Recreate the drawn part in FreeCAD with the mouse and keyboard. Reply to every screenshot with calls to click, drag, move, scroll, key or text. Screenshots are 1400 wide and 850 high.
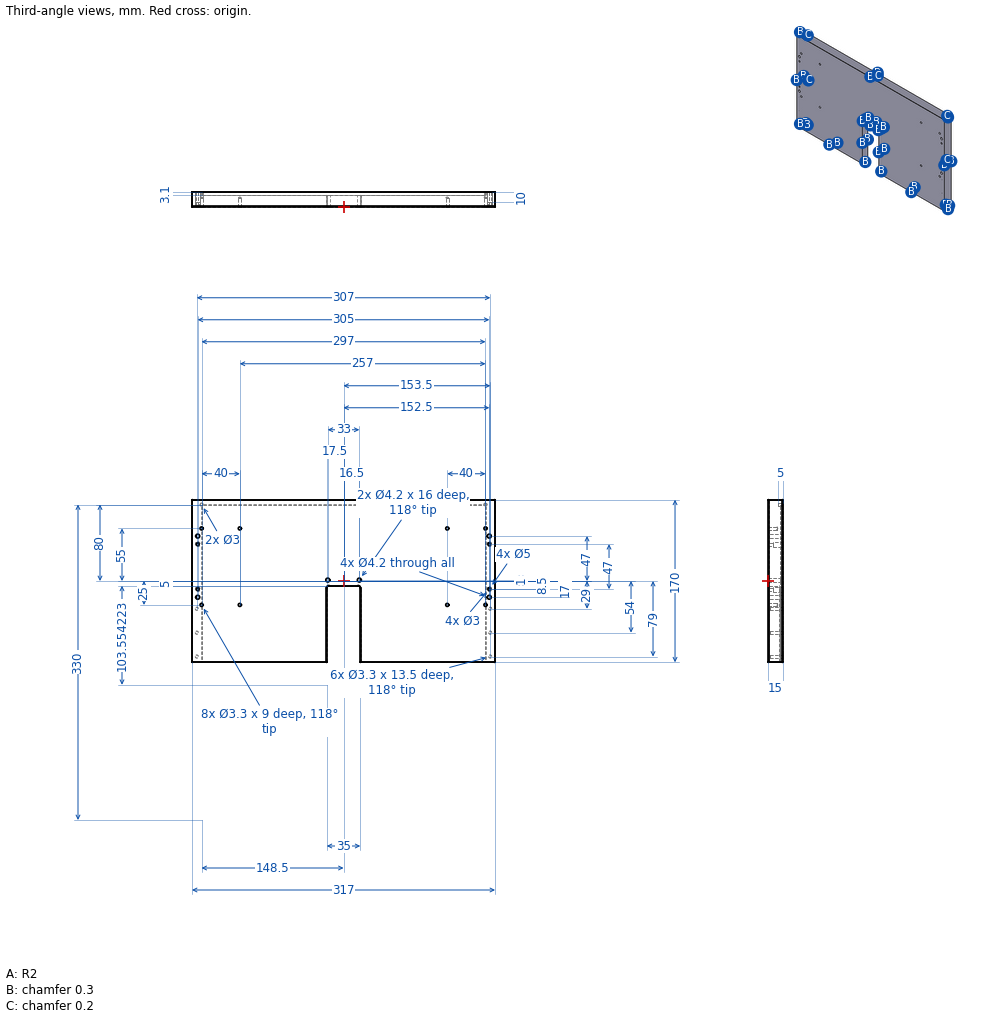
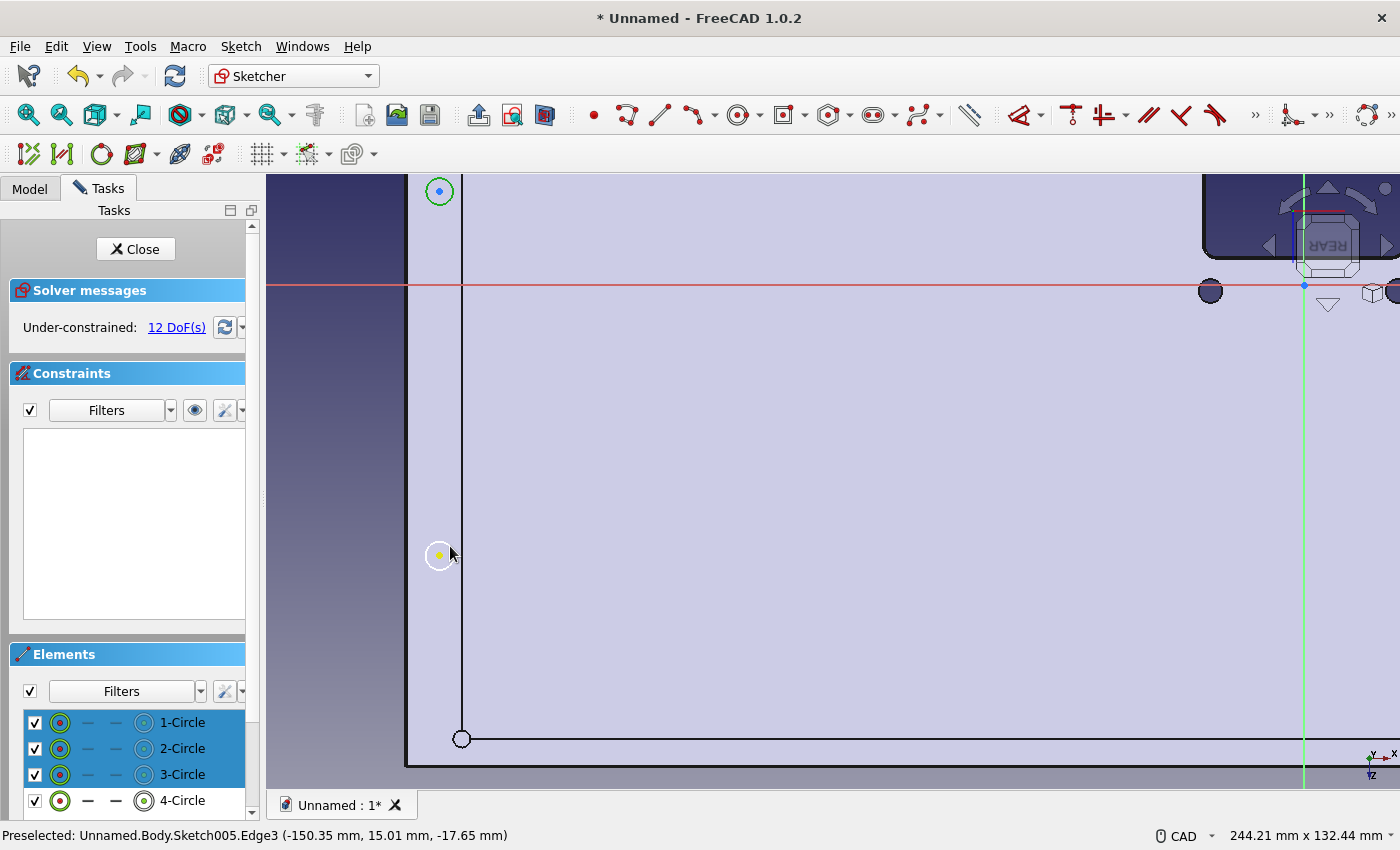
click(450, 546)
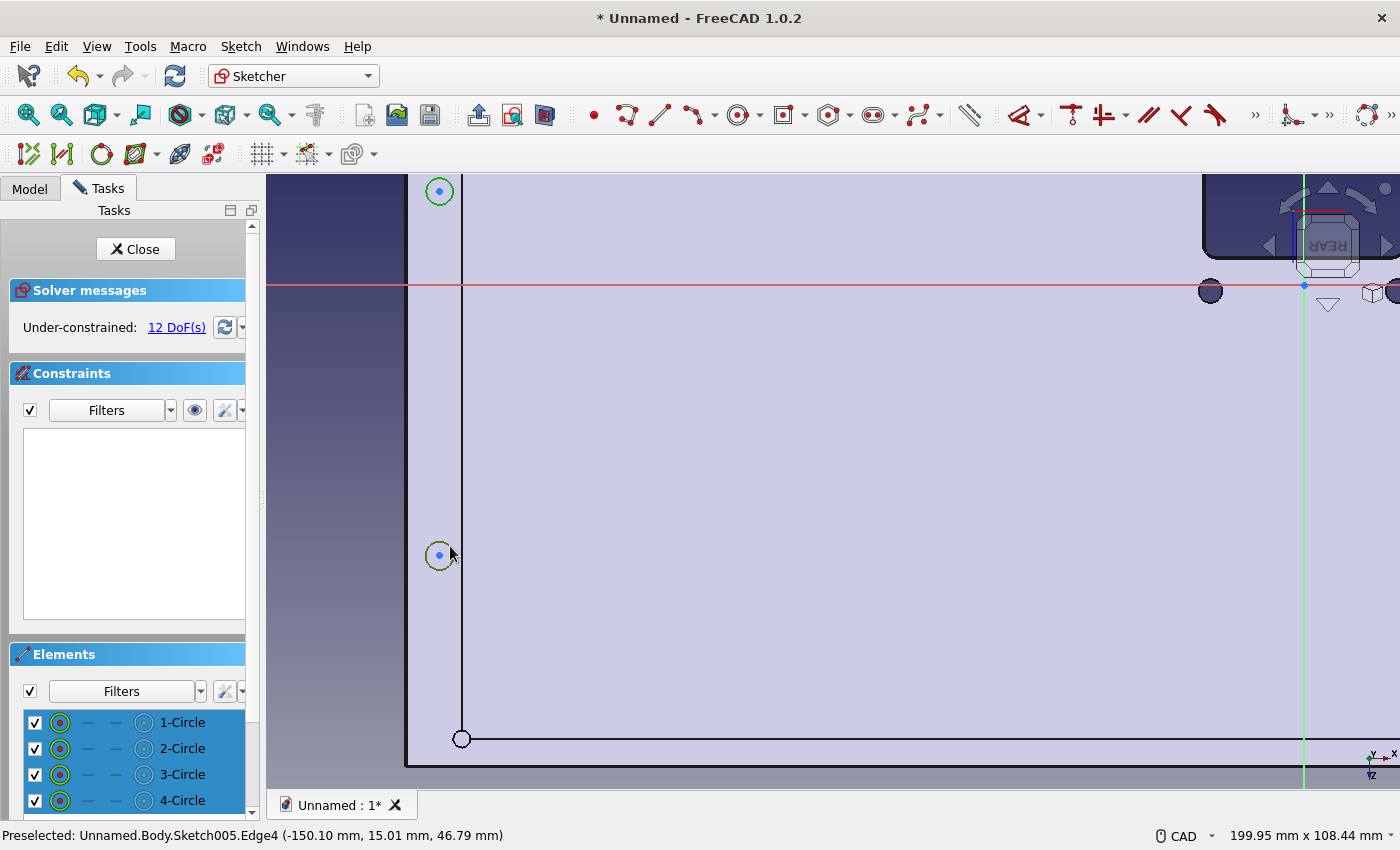
key(e)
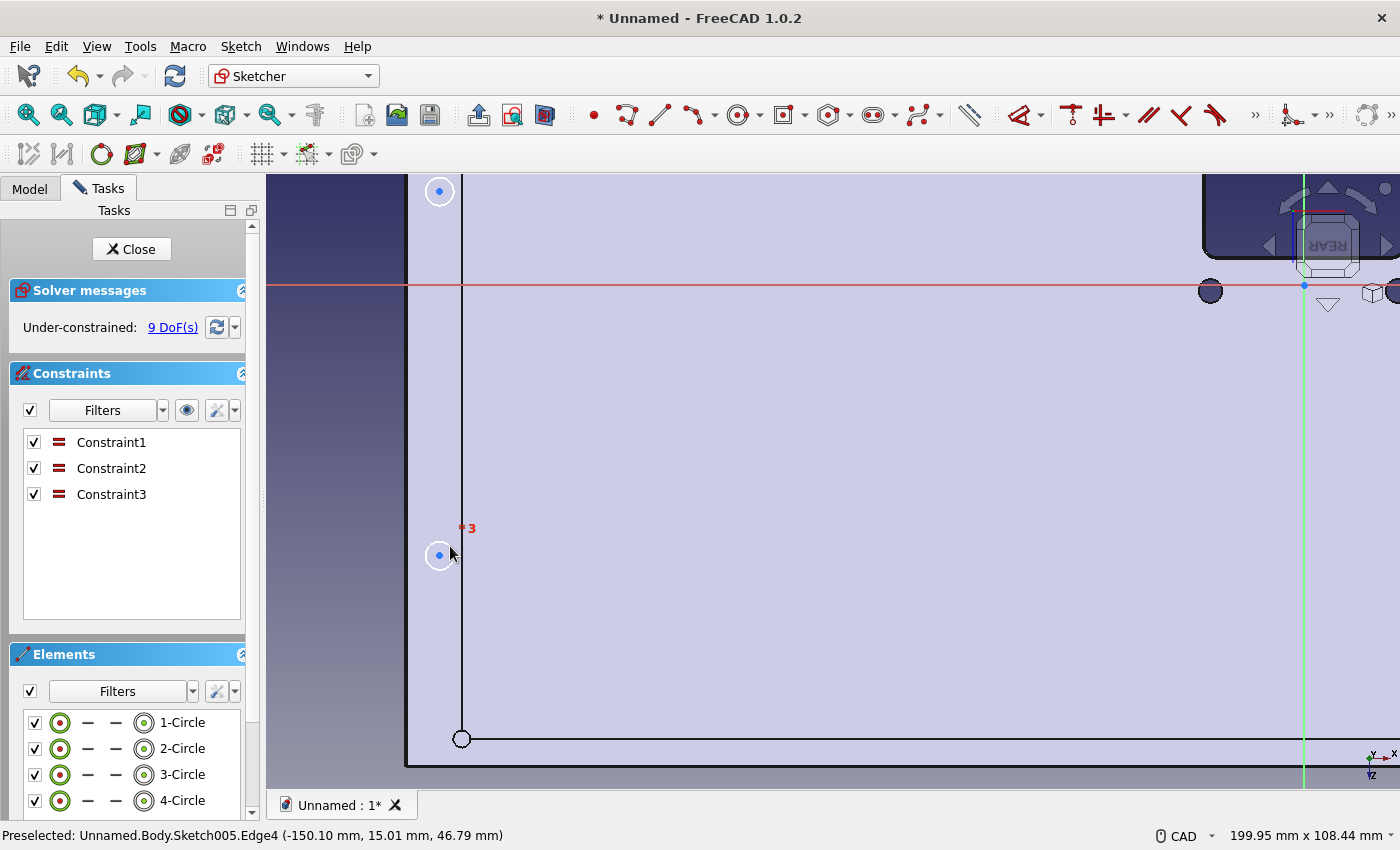
scroll(450, 546, down, 5)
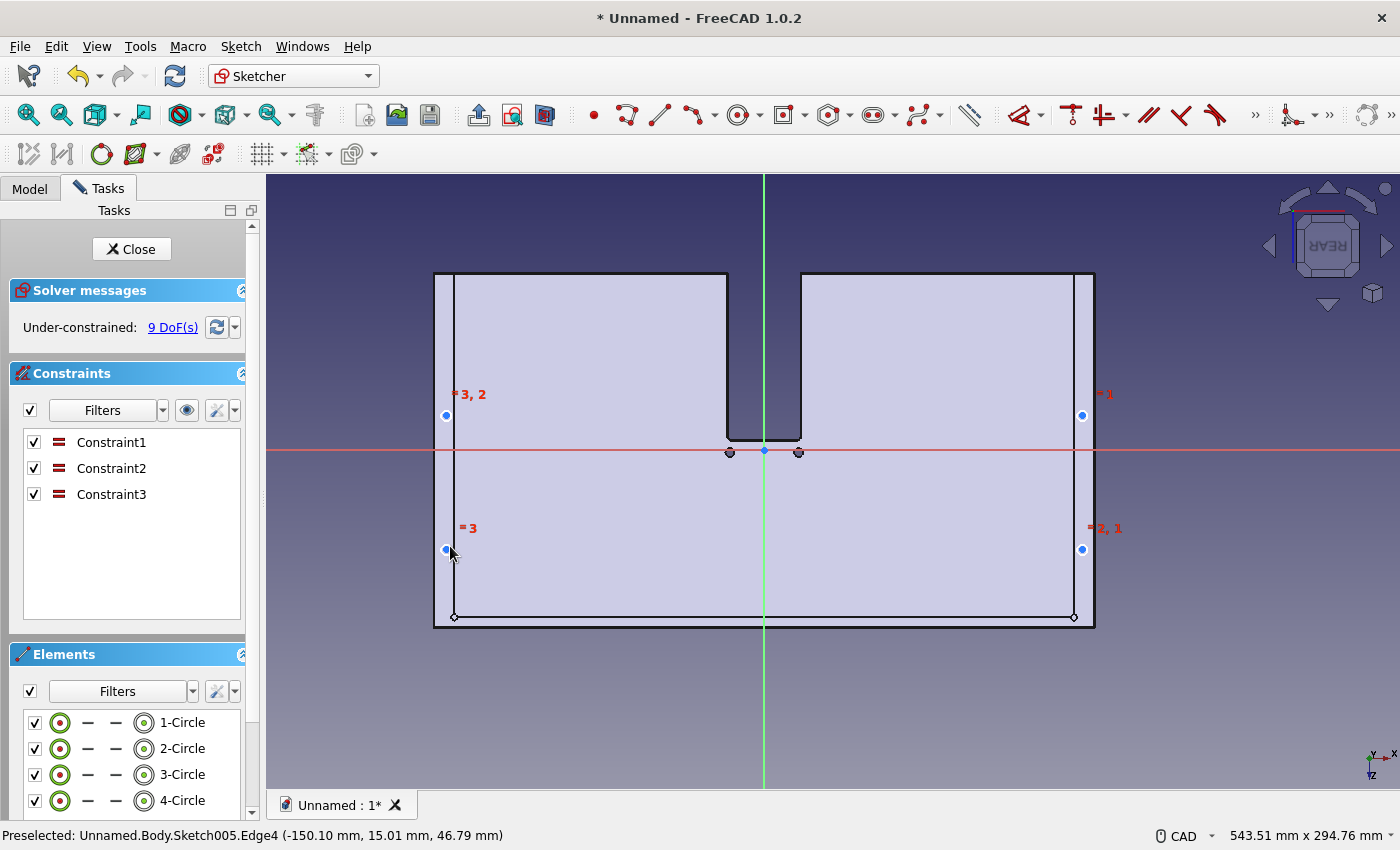
click(1082, 416)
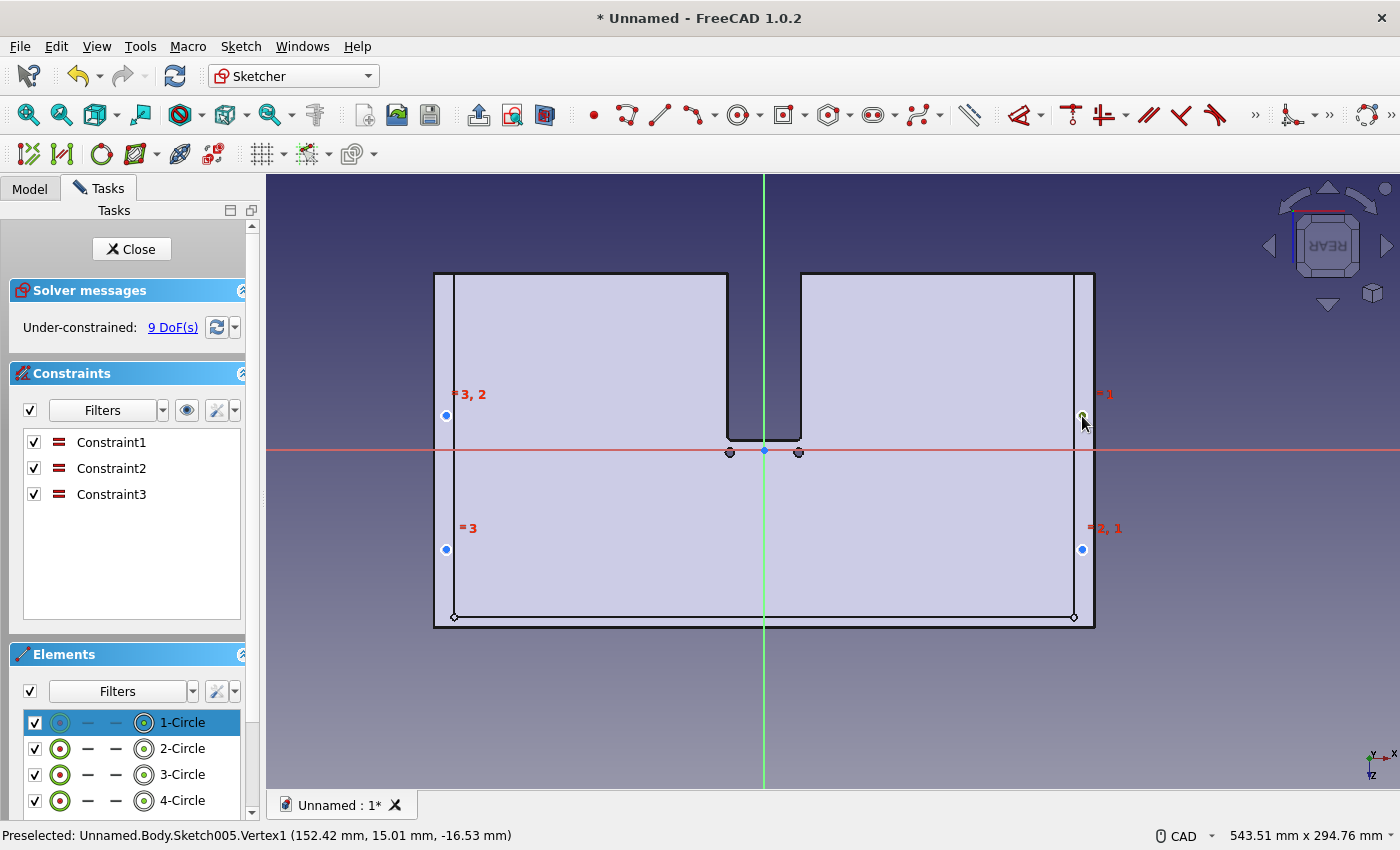
click(1082, 550)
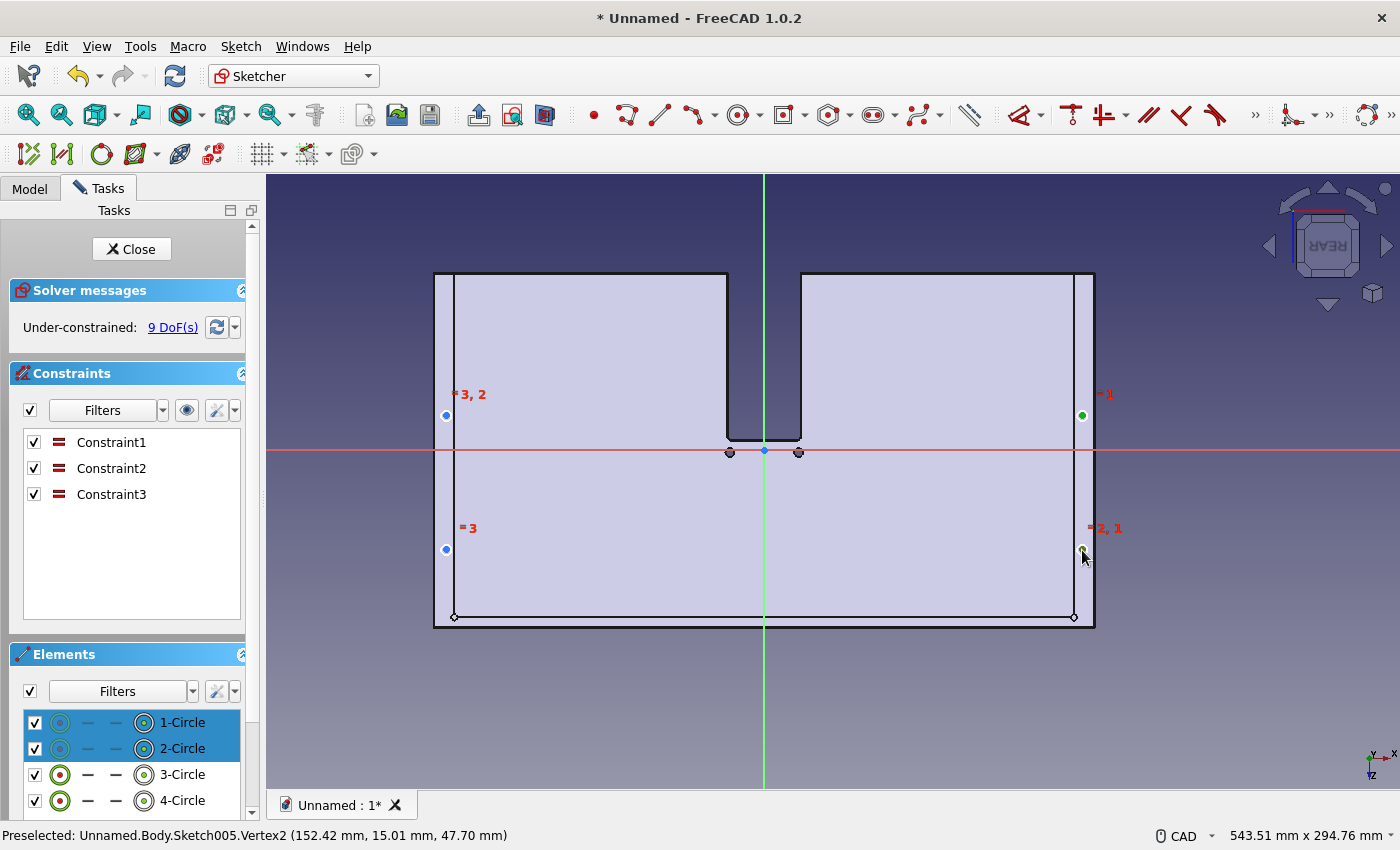
key(v)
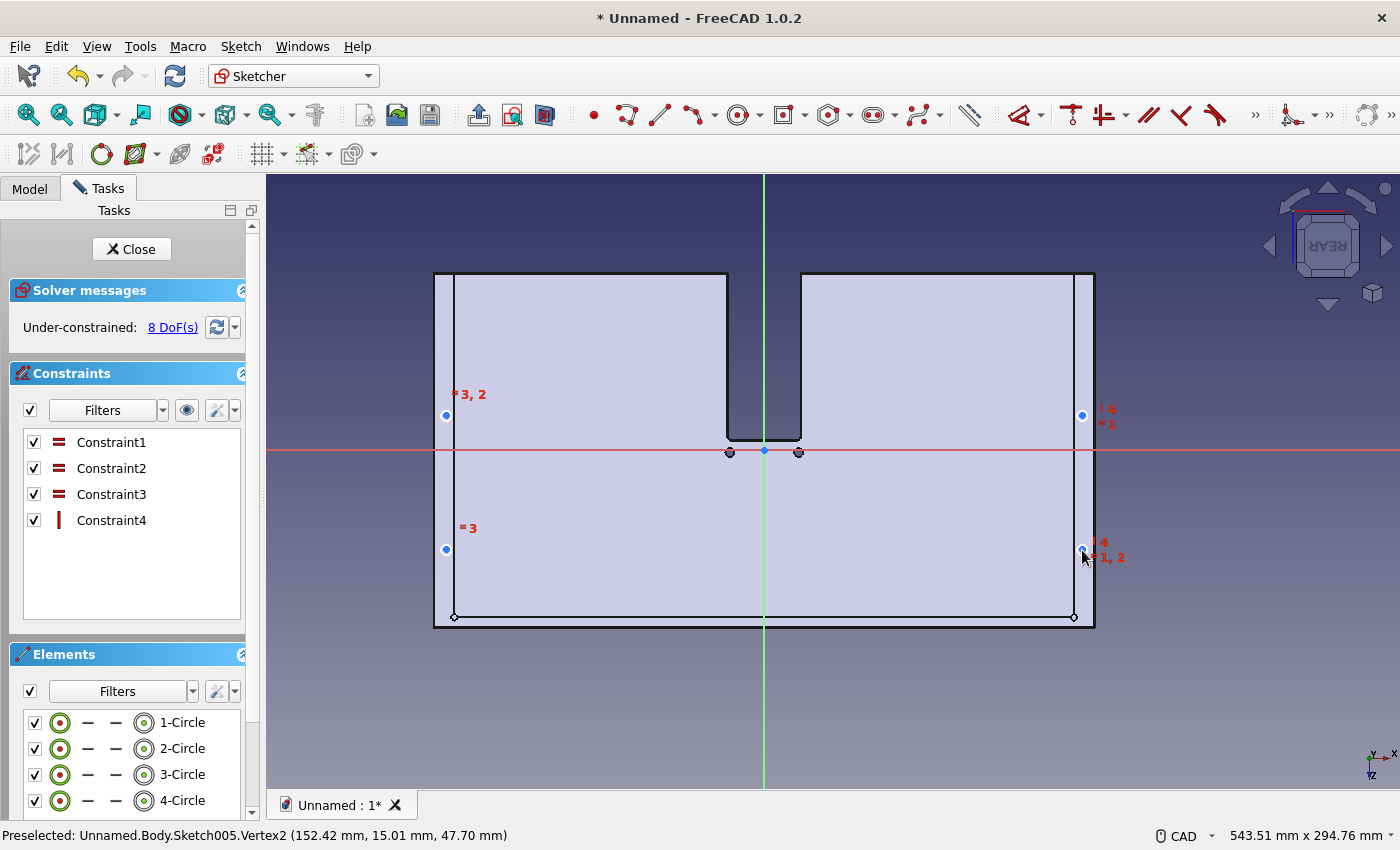
click(1082, 416)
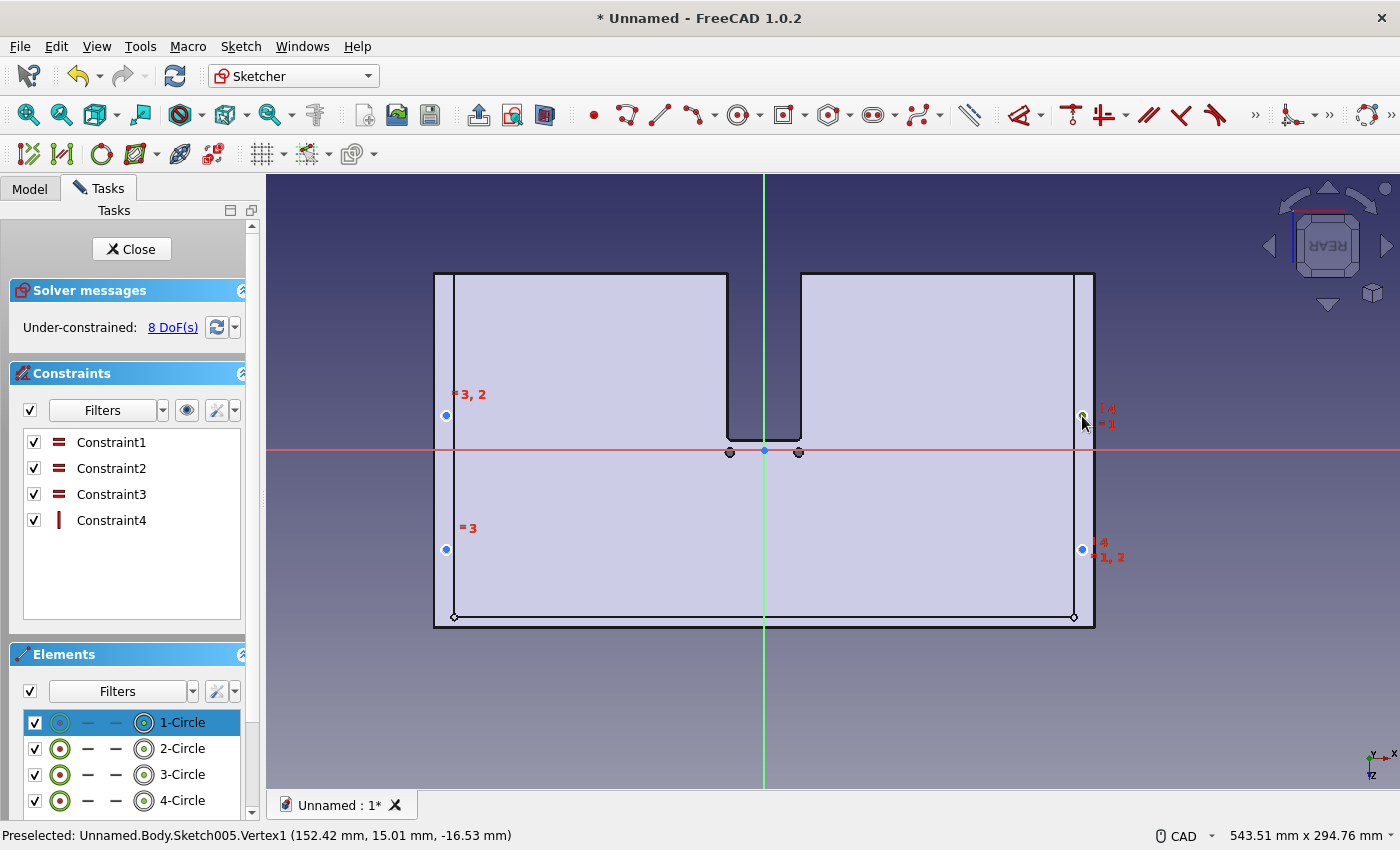
click(446, 416)